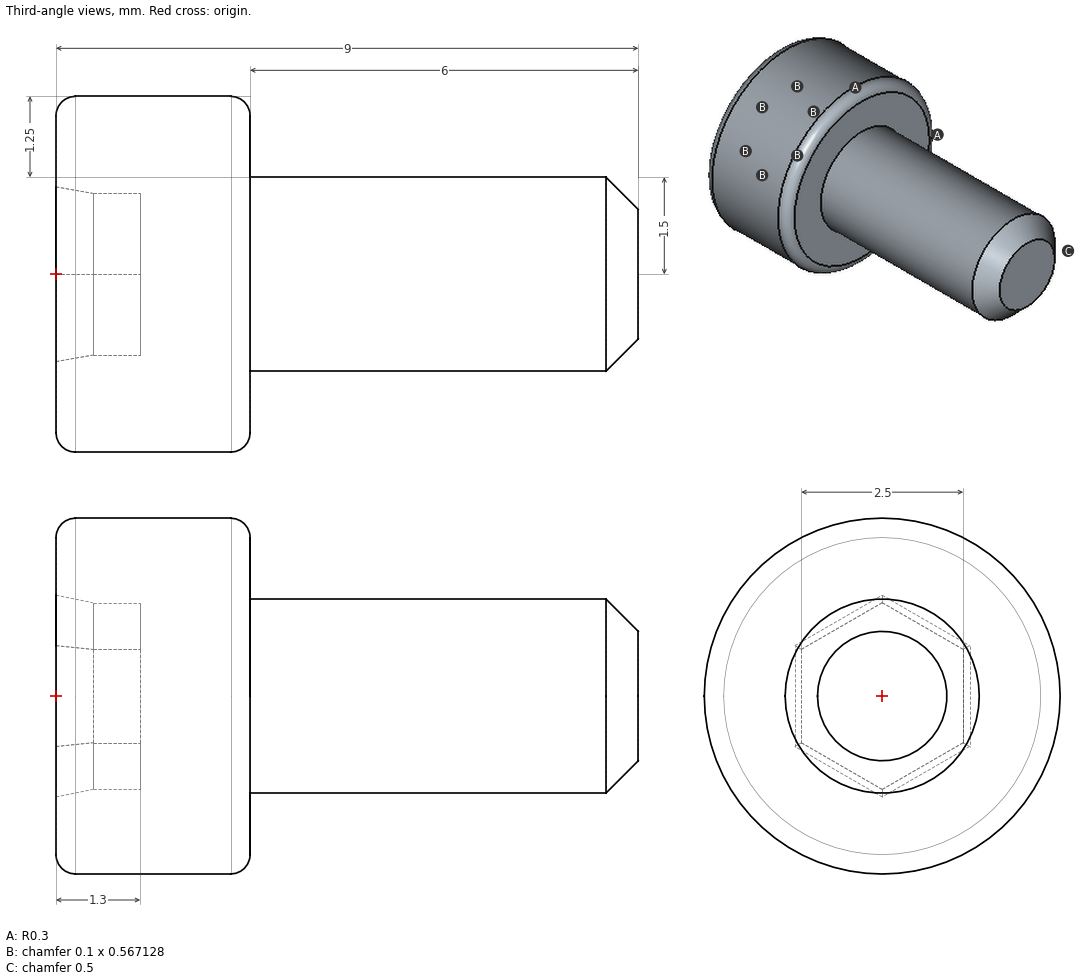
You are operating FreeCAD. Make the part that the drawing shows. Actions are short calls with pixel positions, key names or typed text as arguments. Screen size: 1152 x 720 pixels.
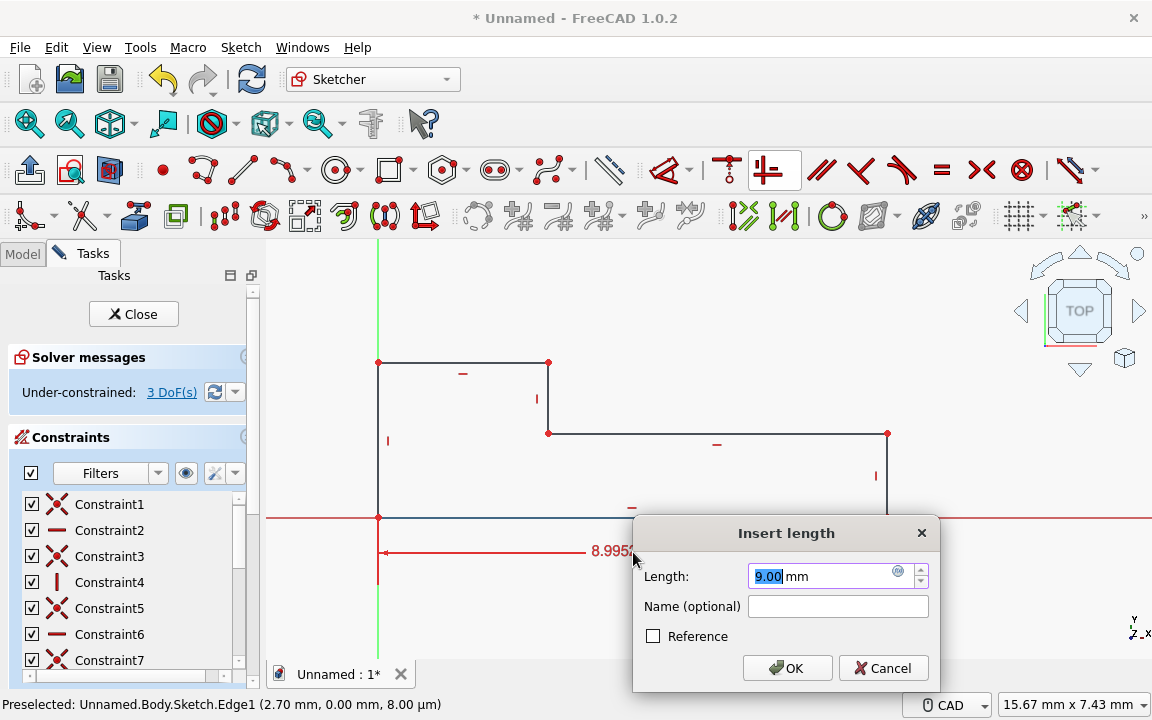
text(9)
key(Return)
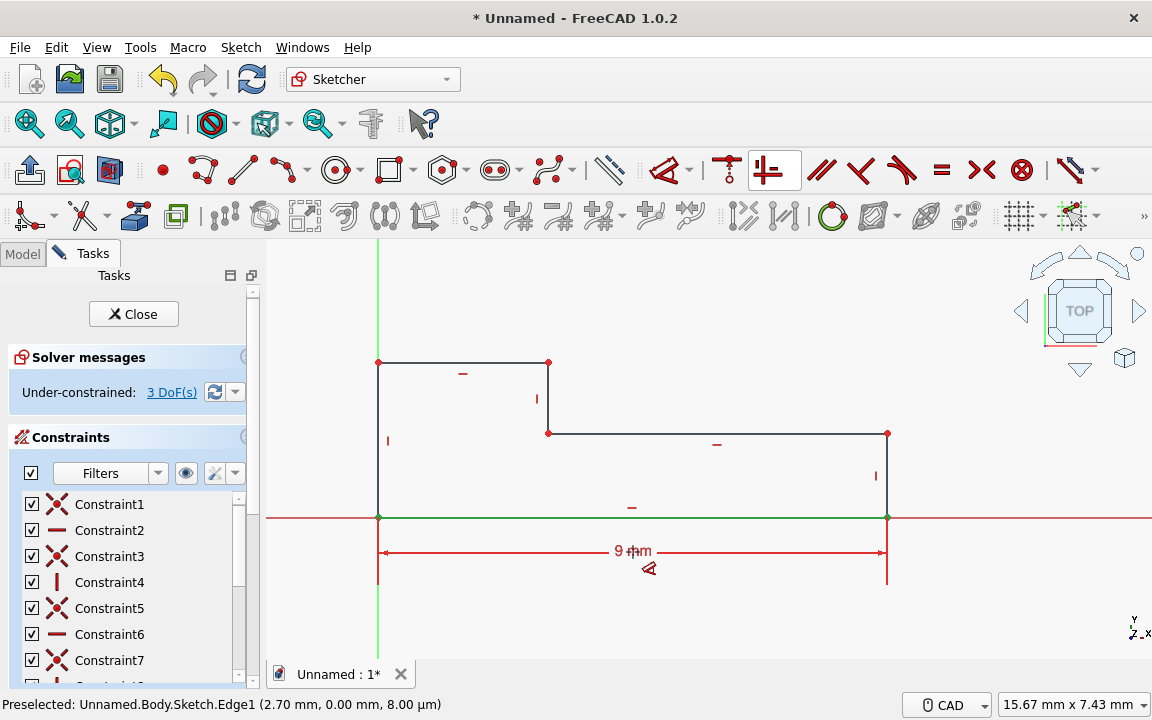
click(785, 434)
click(718, 400)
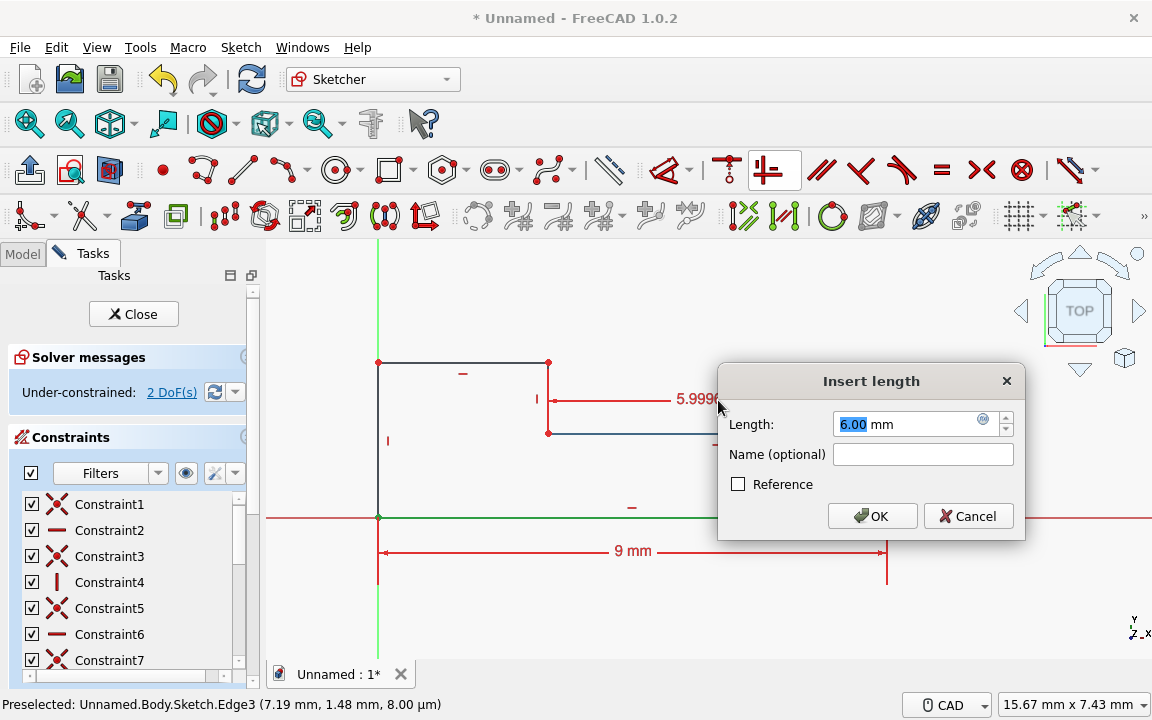
text(6)
key(Return)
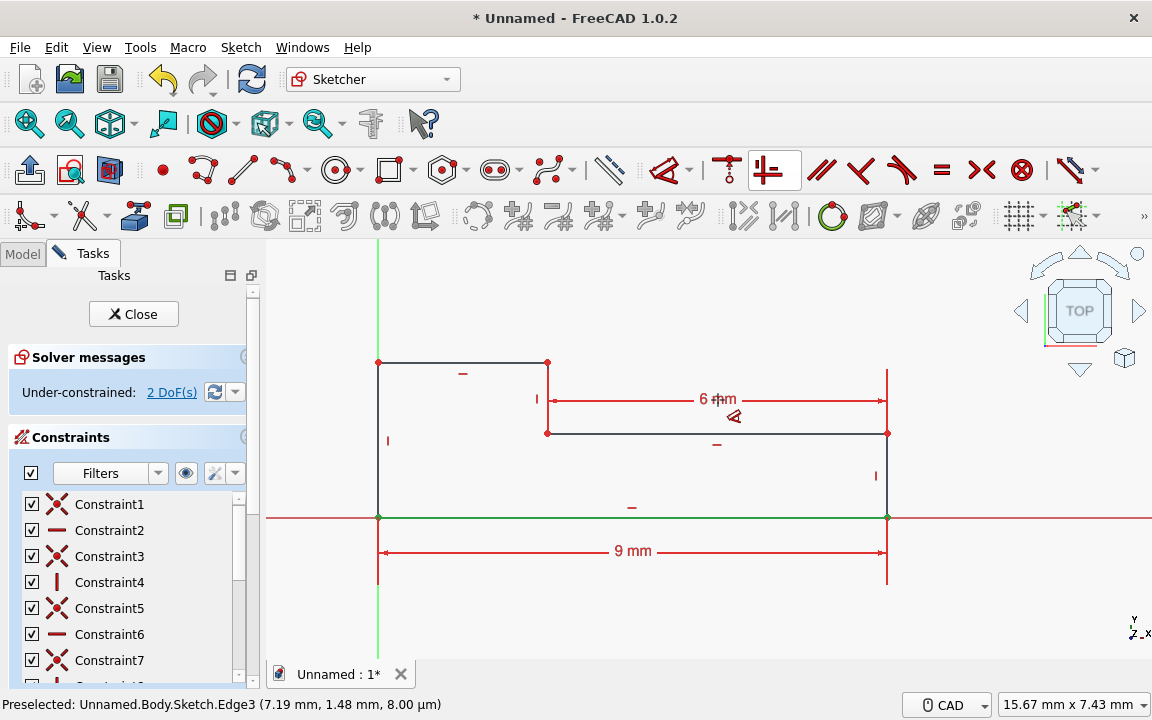
click(887, 493)
click(921, 476)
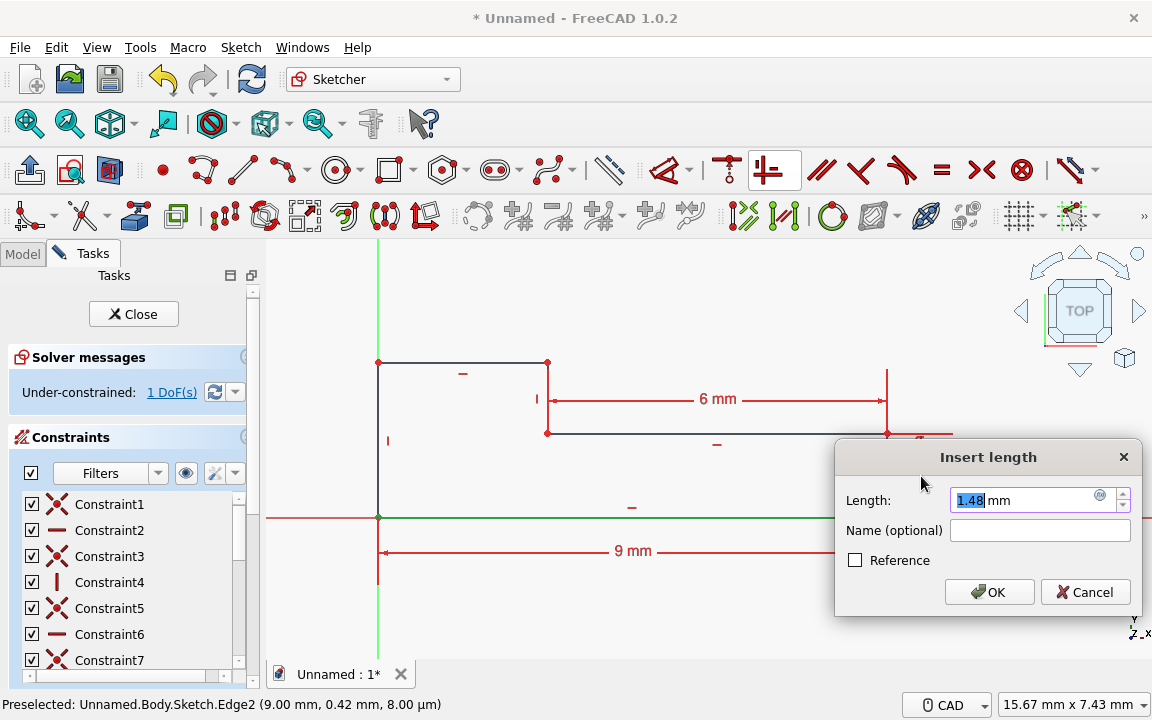
text(1.5)
key(Return)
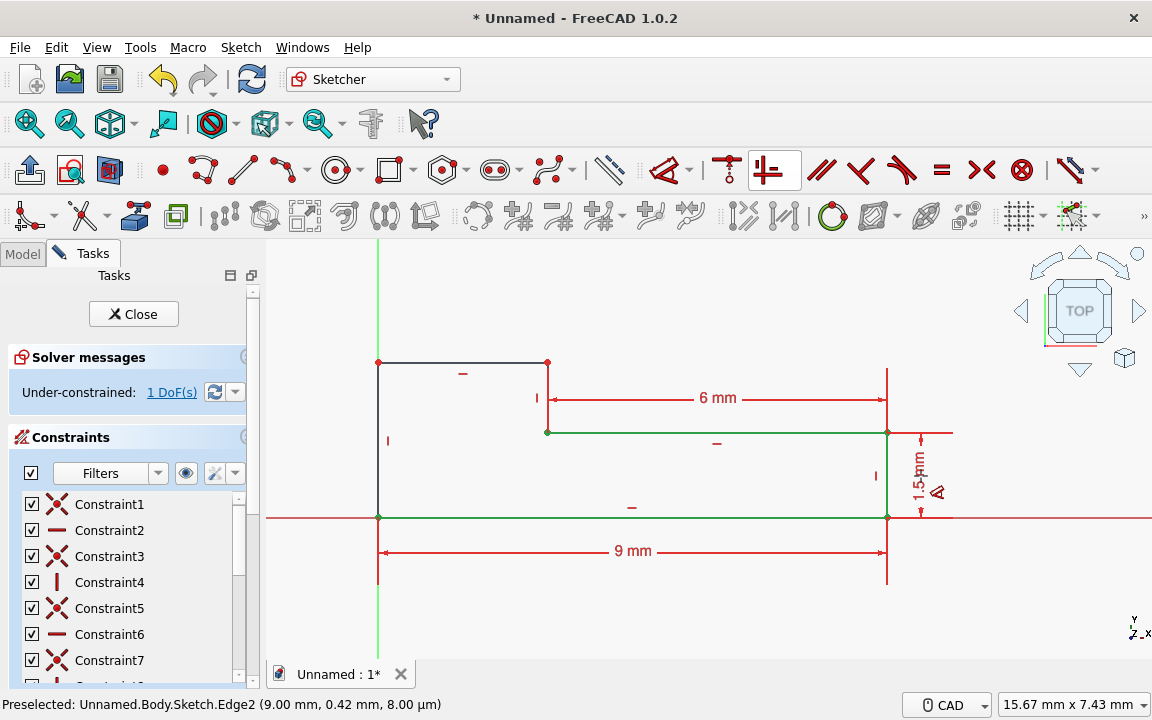
click(548, 412)
click(514, 398)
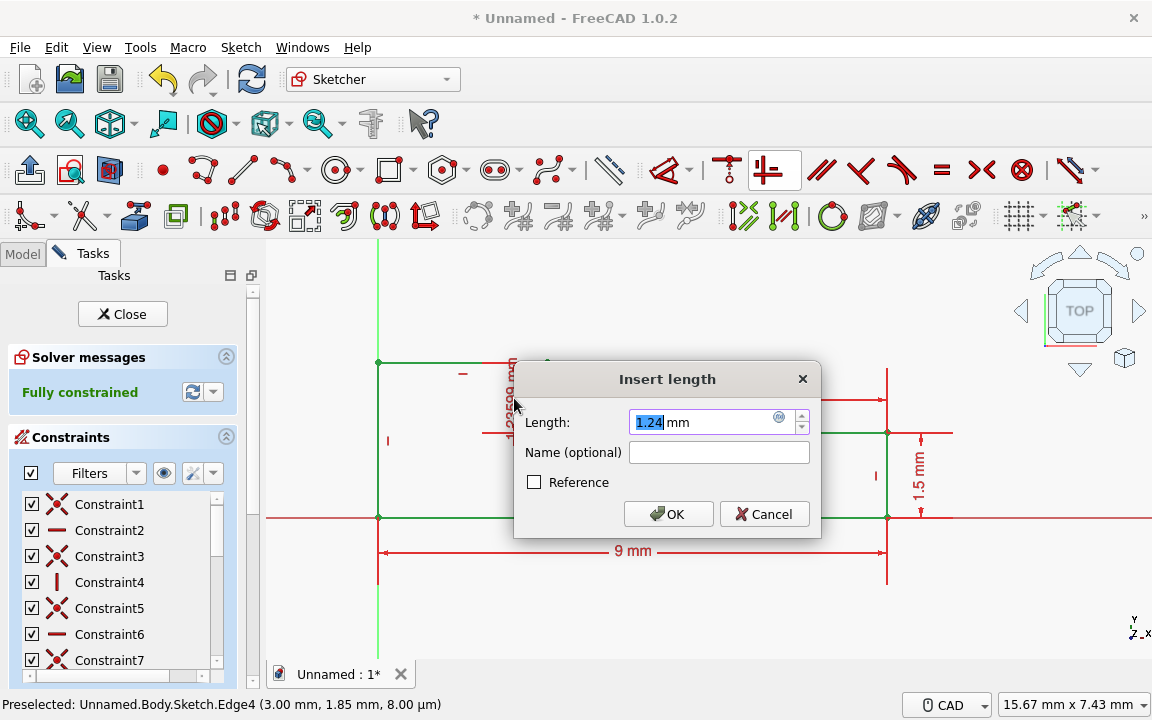
text(1.25)
key(Return)
key(Escape)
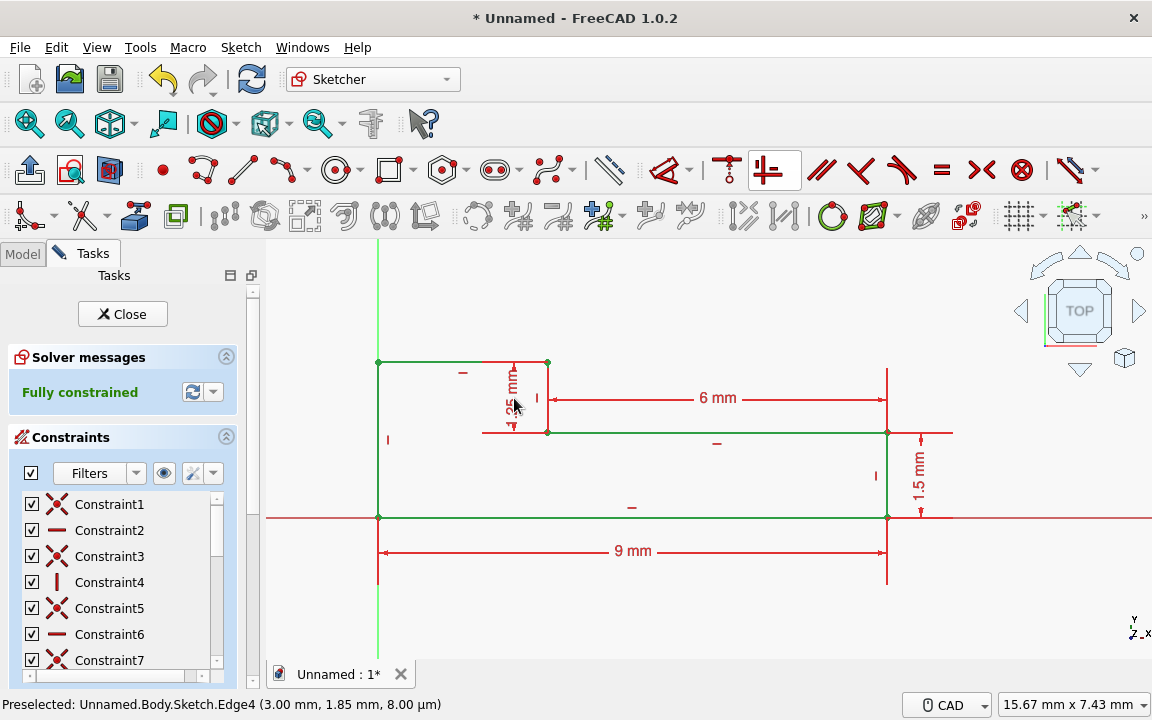
click(123, 314)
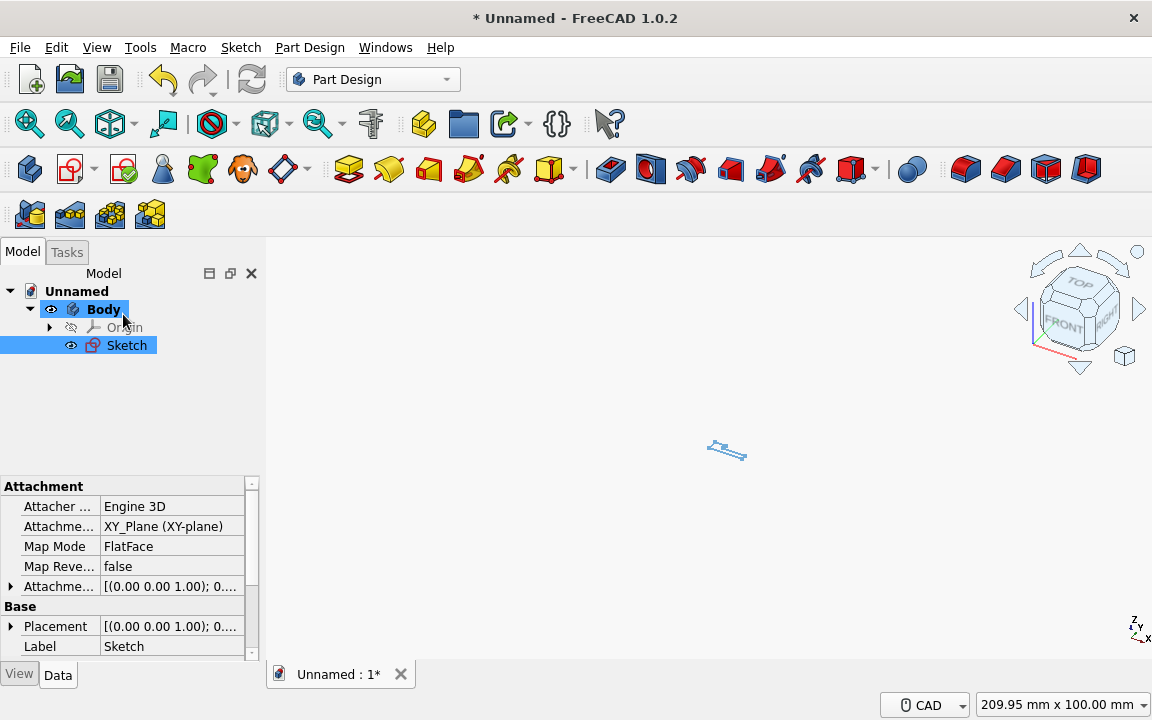
click(390, 170)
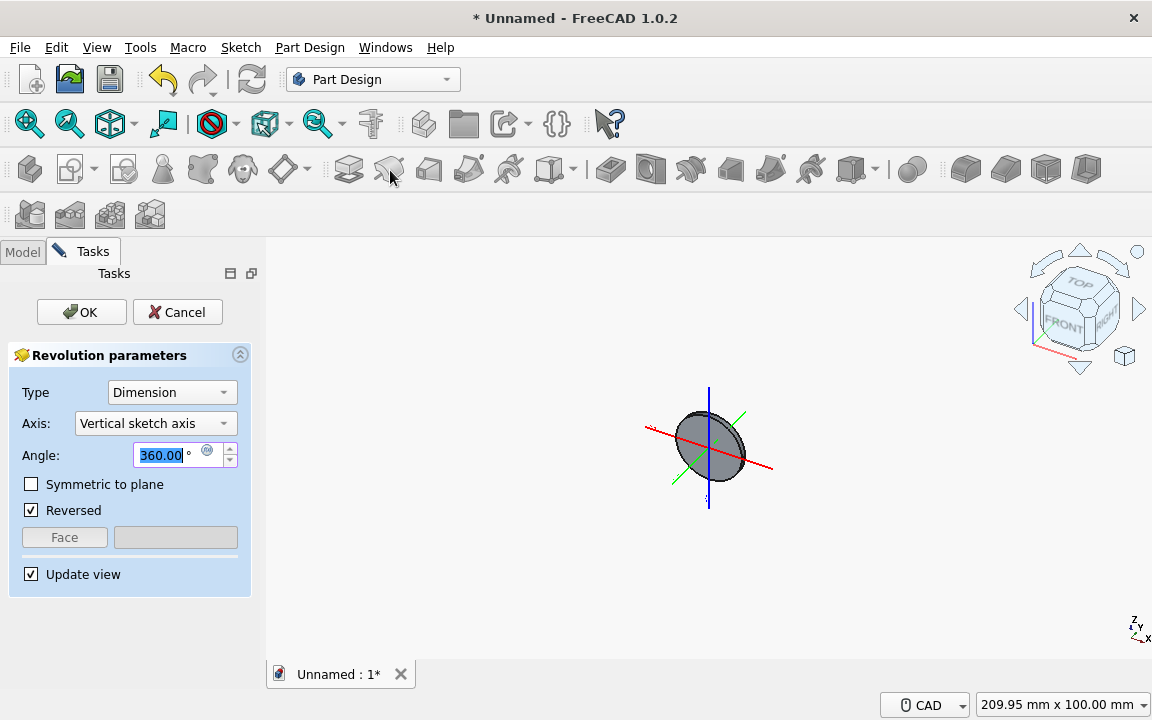
click(156, 424)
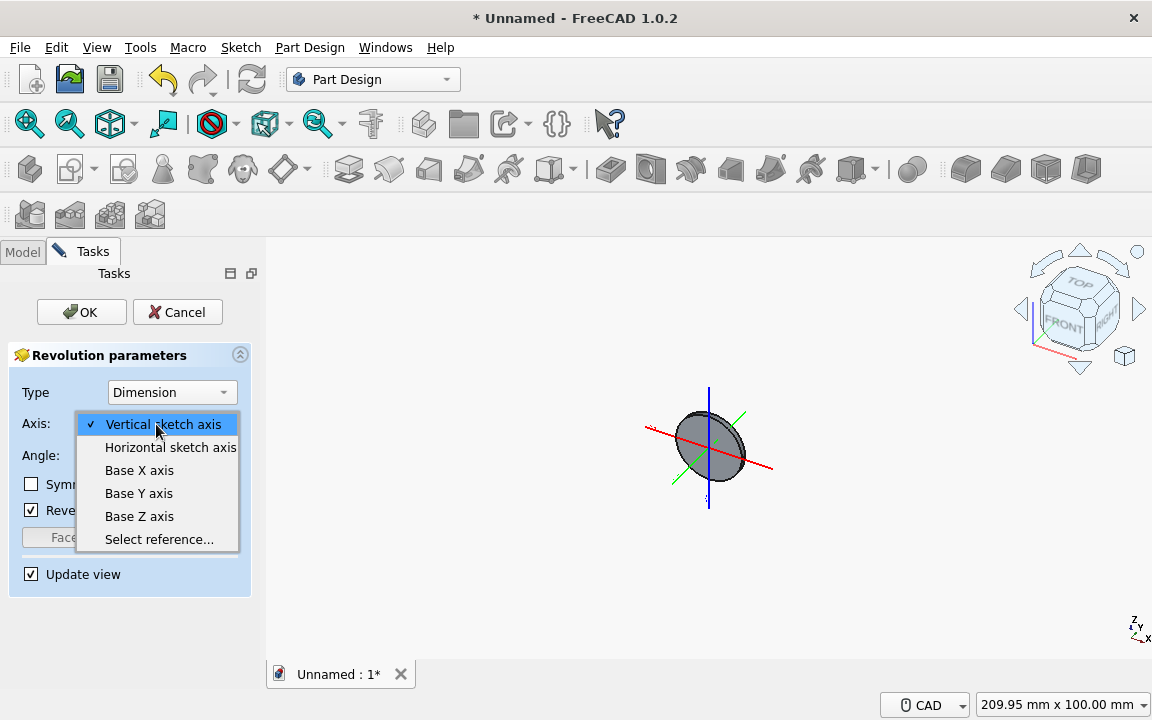
click(156, 448)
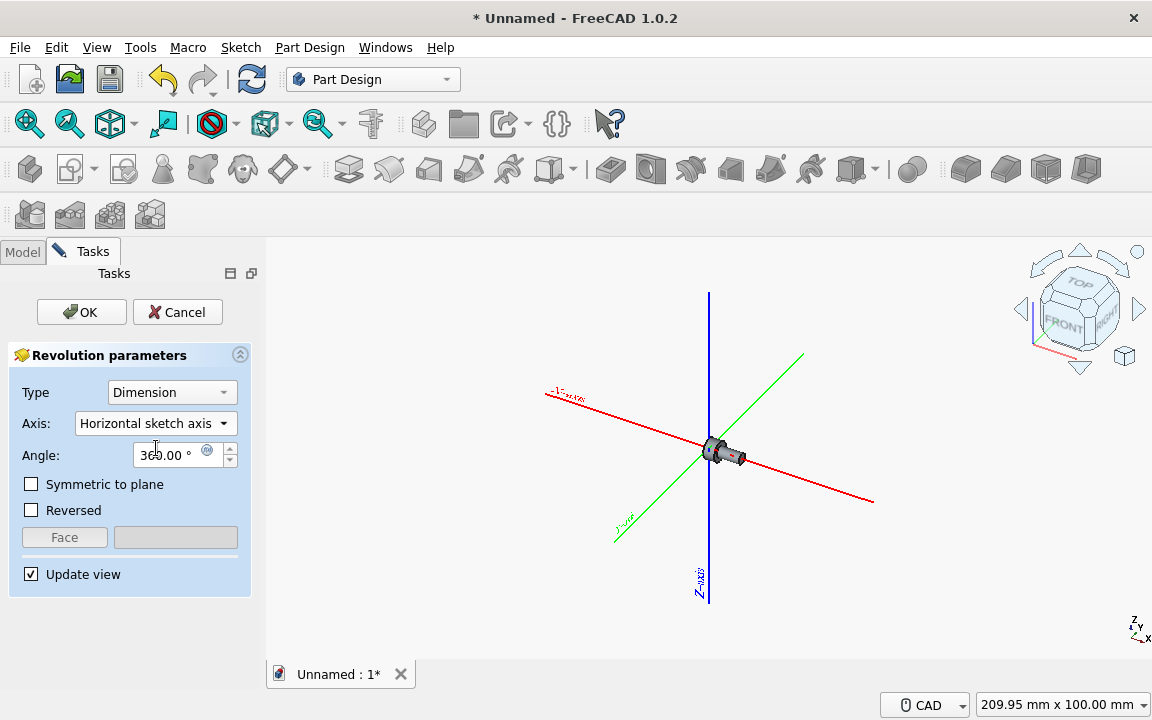
click(82, 312)